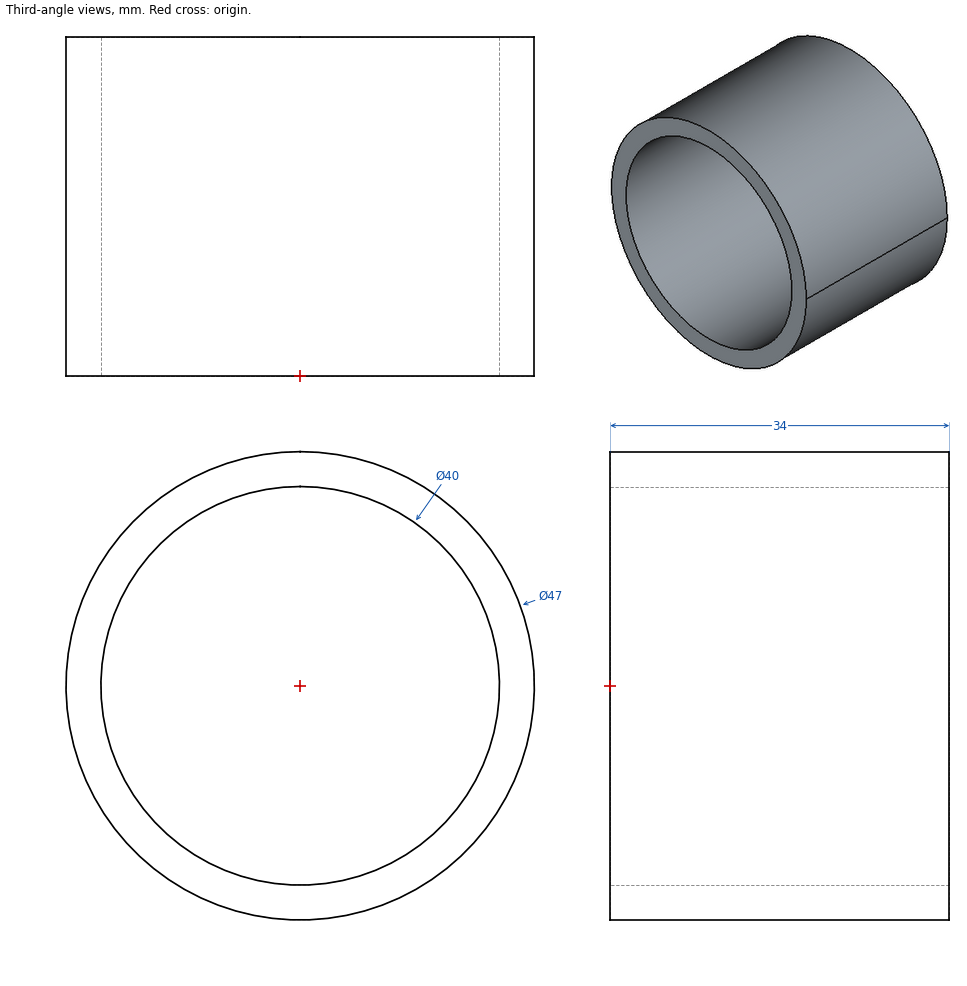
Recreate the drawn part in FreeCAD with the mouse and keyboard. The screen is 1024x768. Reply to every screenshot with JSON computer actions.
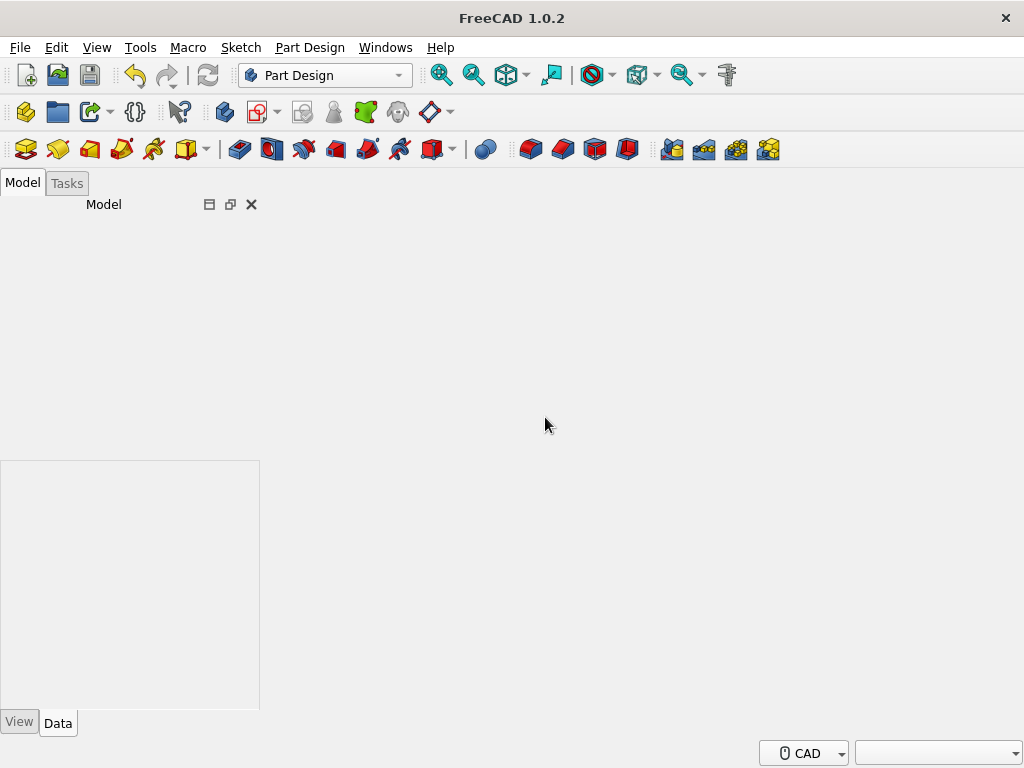
{"action": "left_click", "coordinate": [26, 76]}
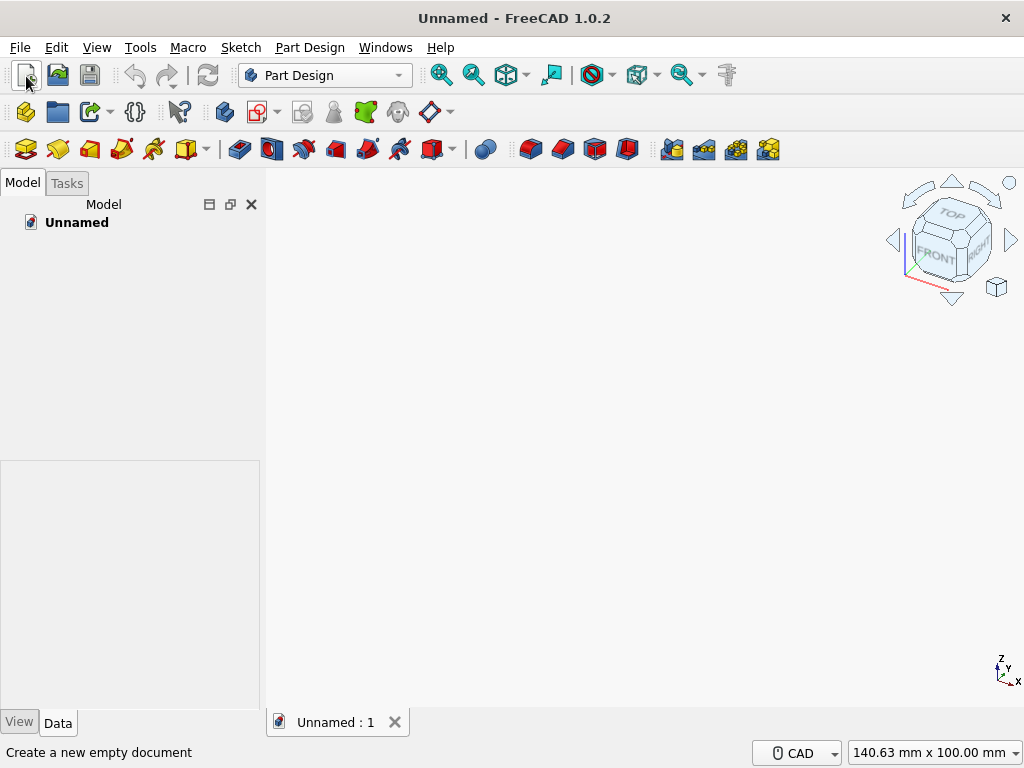
{"action": "left_click", "coordinate": [258, 112]}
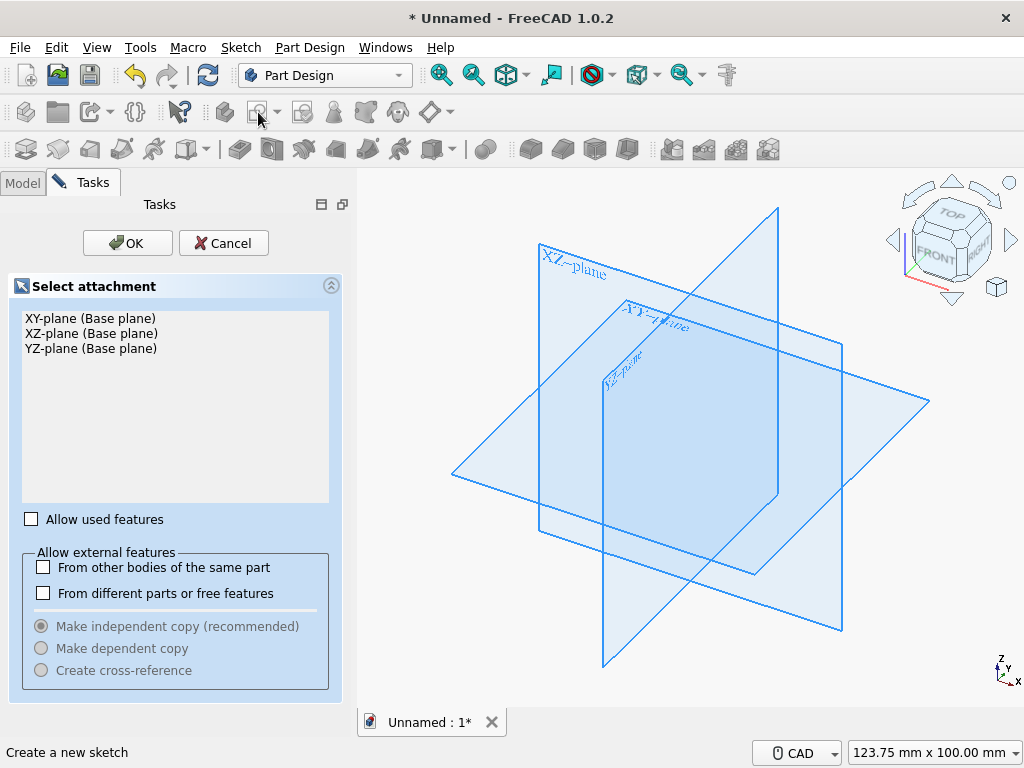
{"action": "left_click", "coordinate": [82, 334]}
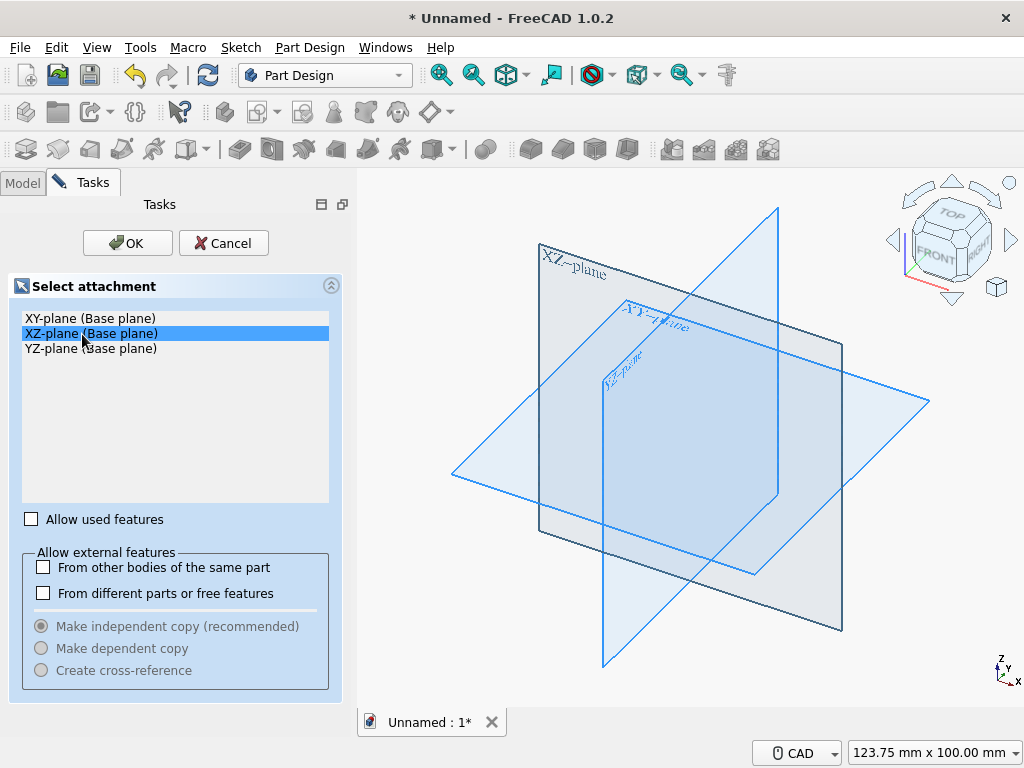
{"action": "left_click", "coordinate": [128, 243]}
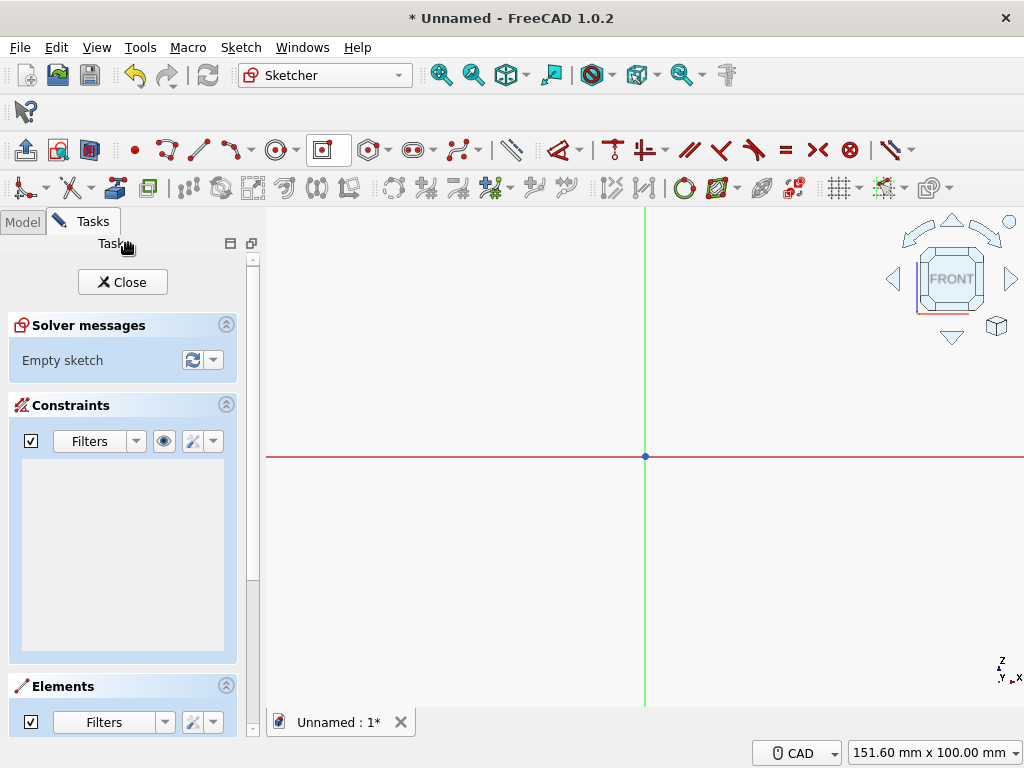
{"action": "left_click", "coordinate": [276, 150]}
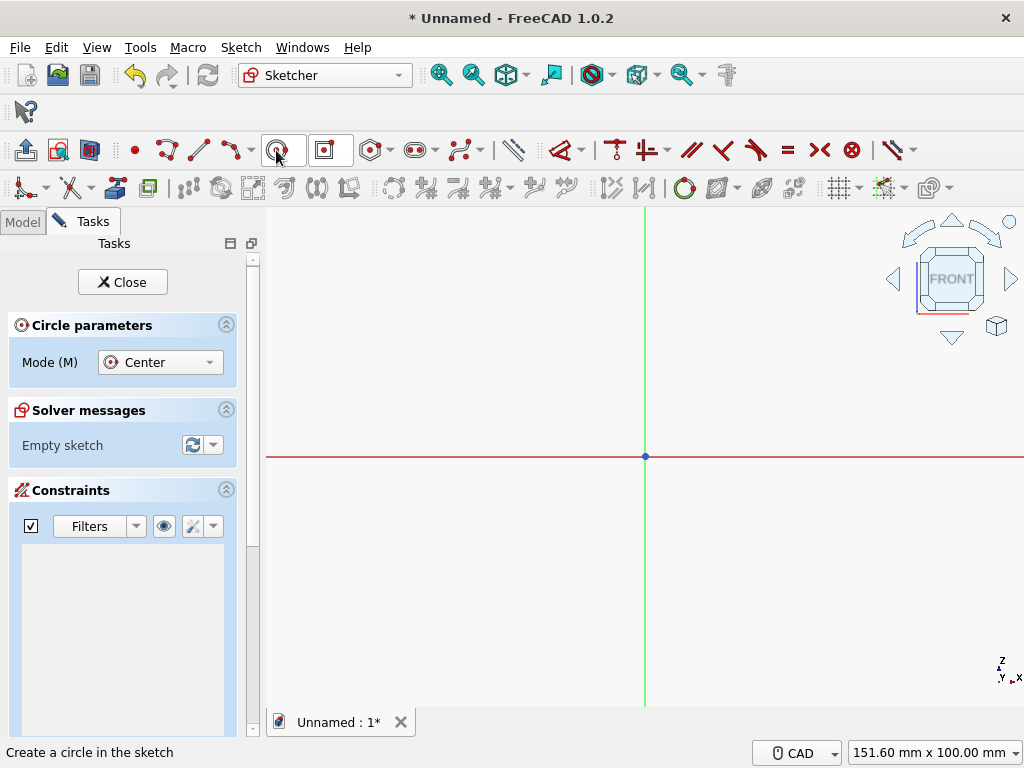
{"action": "left_click", "coordinate": [645, 457]}
{"action": "mouse_move", "coordinate": [728, 374]}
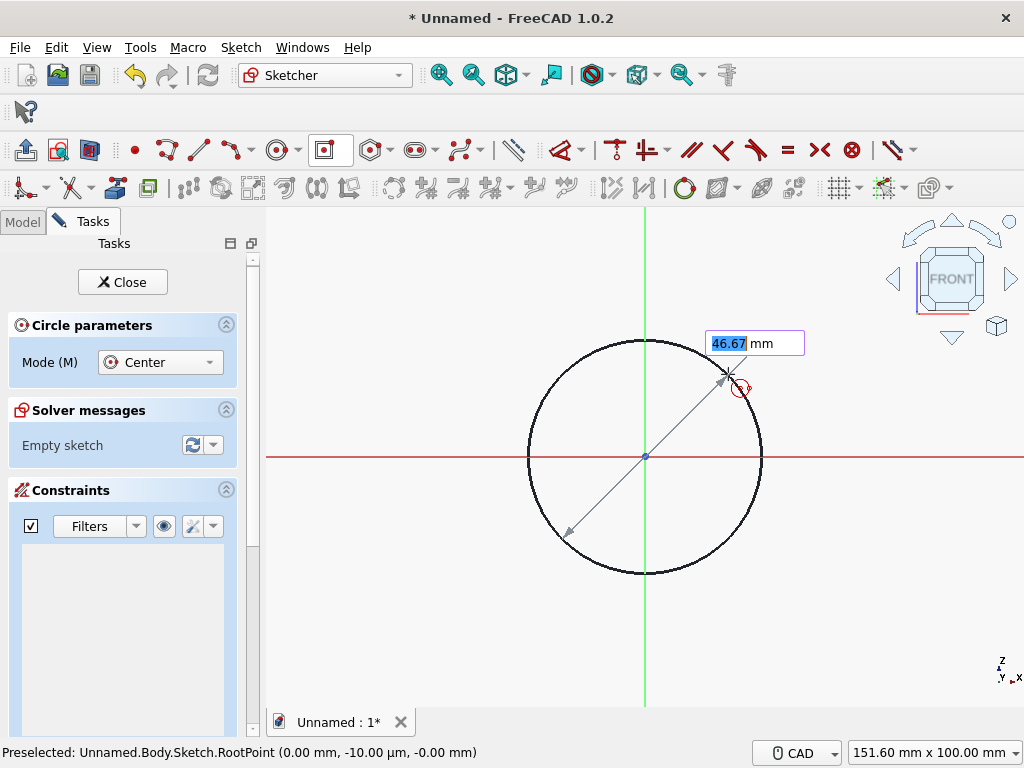
{"action": "type", "text": "47"}
{"action": "key", "text": "Return"}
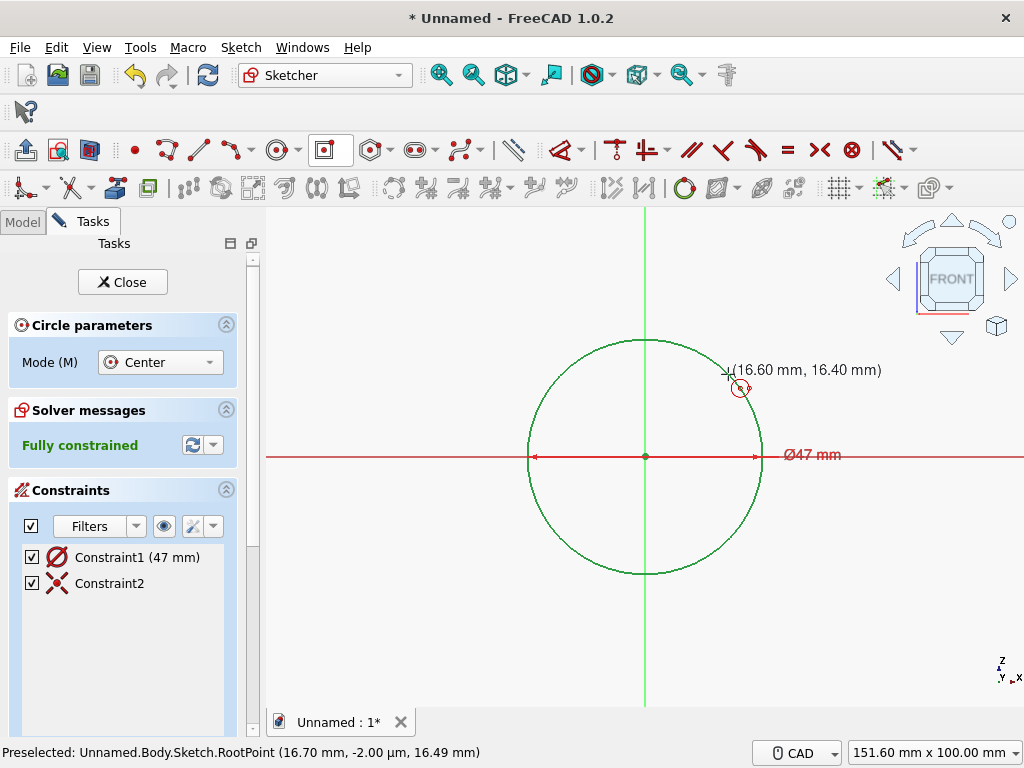
{"action": "left_click", "coordinate": [645, 457]}
{"action": "mouse_move", "coordinate": [716, 386]}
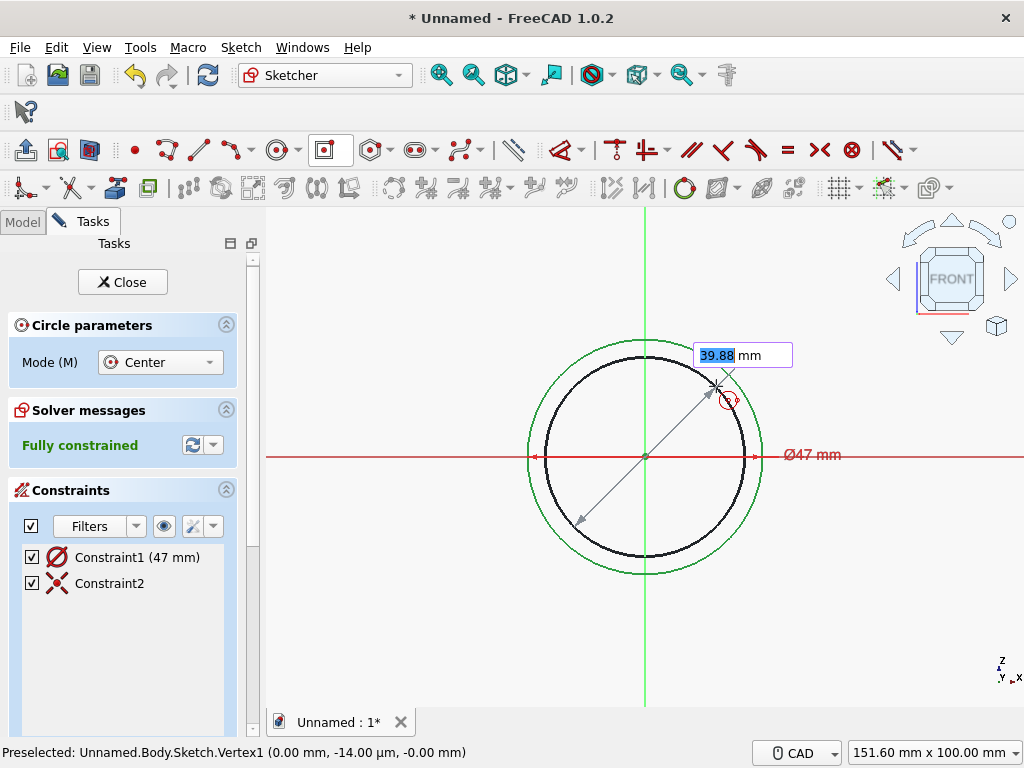
{"action": "type", "text": "40"}
{"action": "key", "text": "Return"}
{"action": "key", "text": "Escape"}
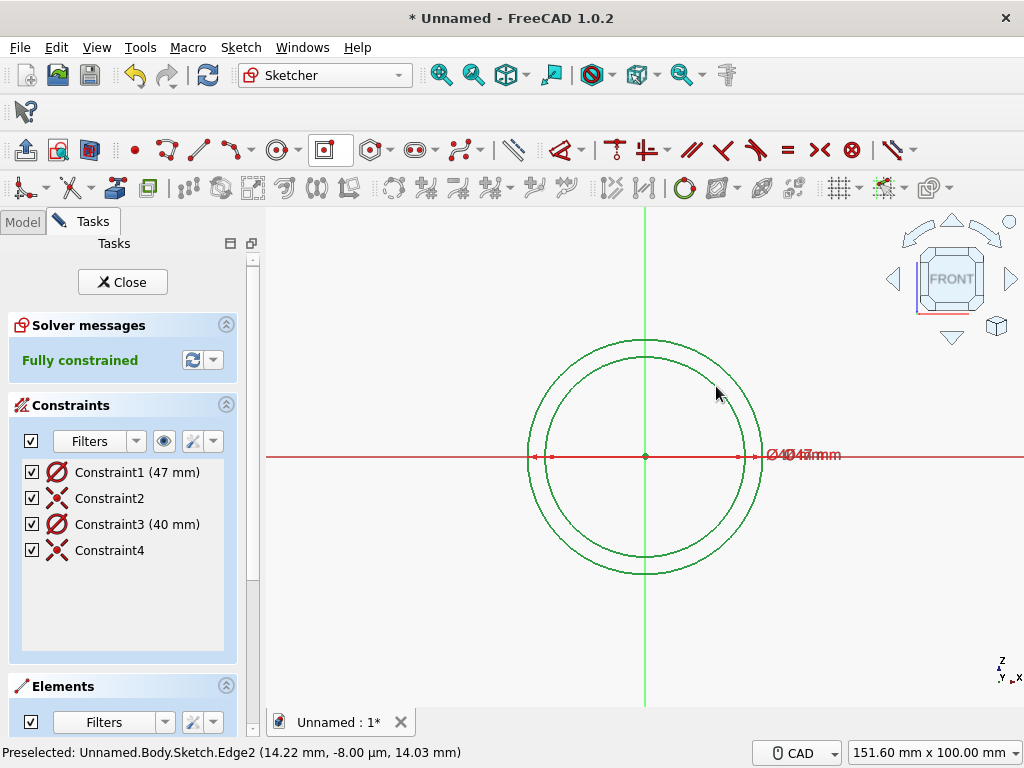
{"action": "left_click", "coordinate": [123, 282]}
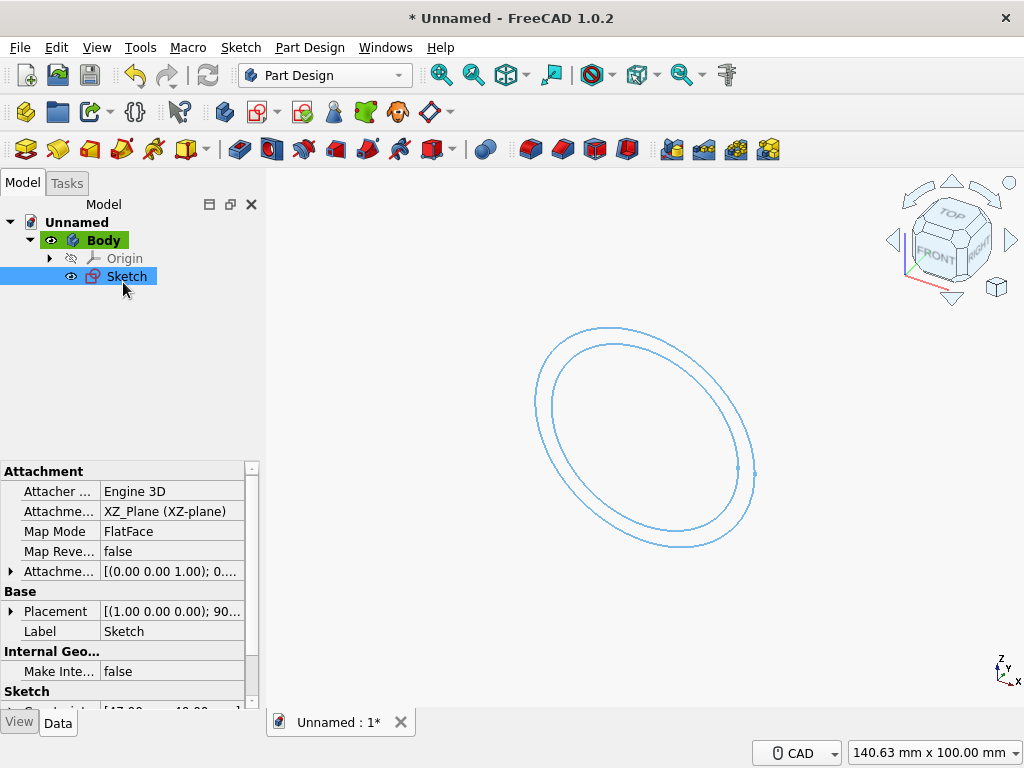
{"action": "left_click", "coordinate": [26, 150]}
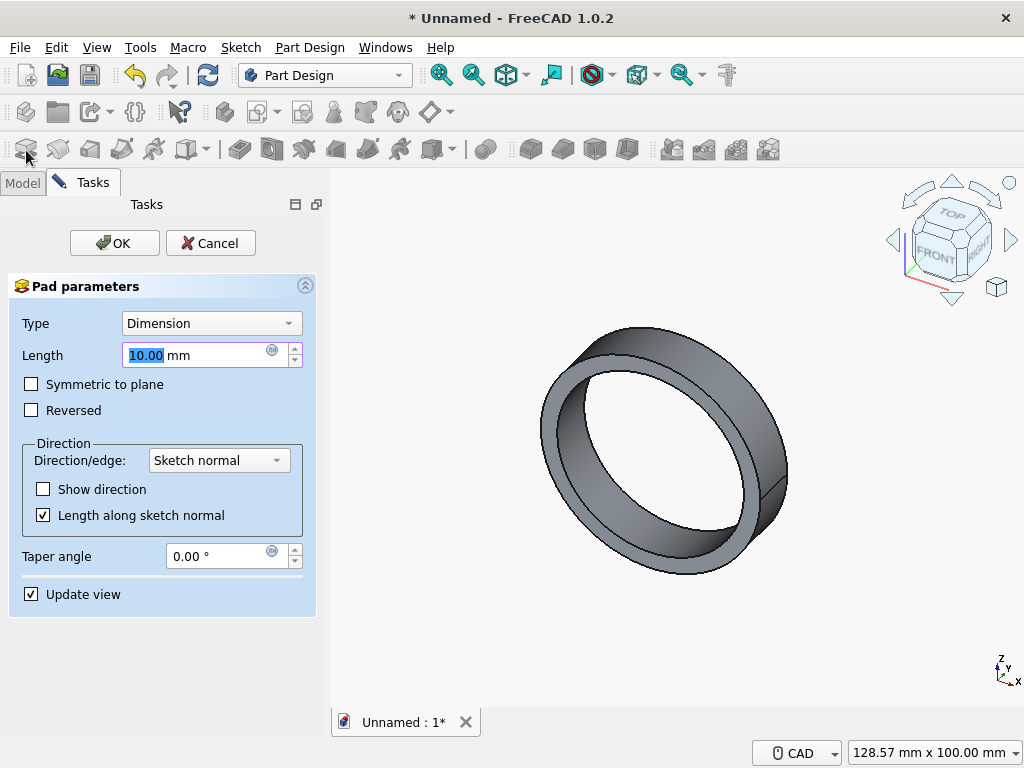
{"action": "type", "text": "34"}
{"action": "key", "text": "Tab"}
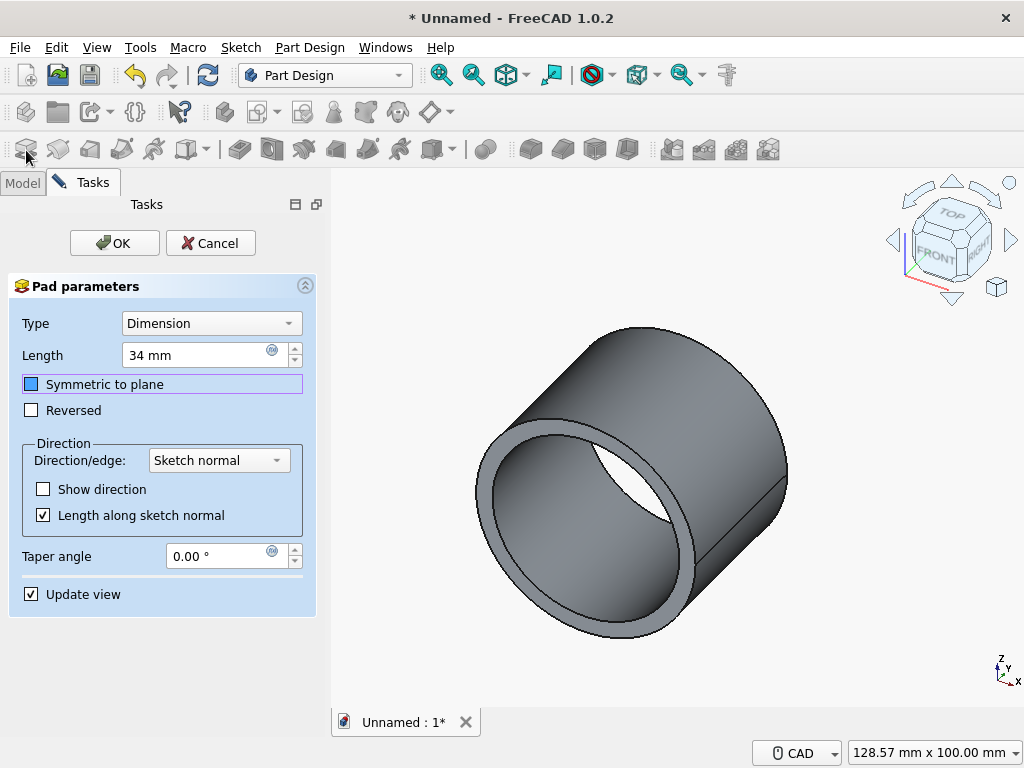
{"action": "left_click", "coordinate": [30, 410]}